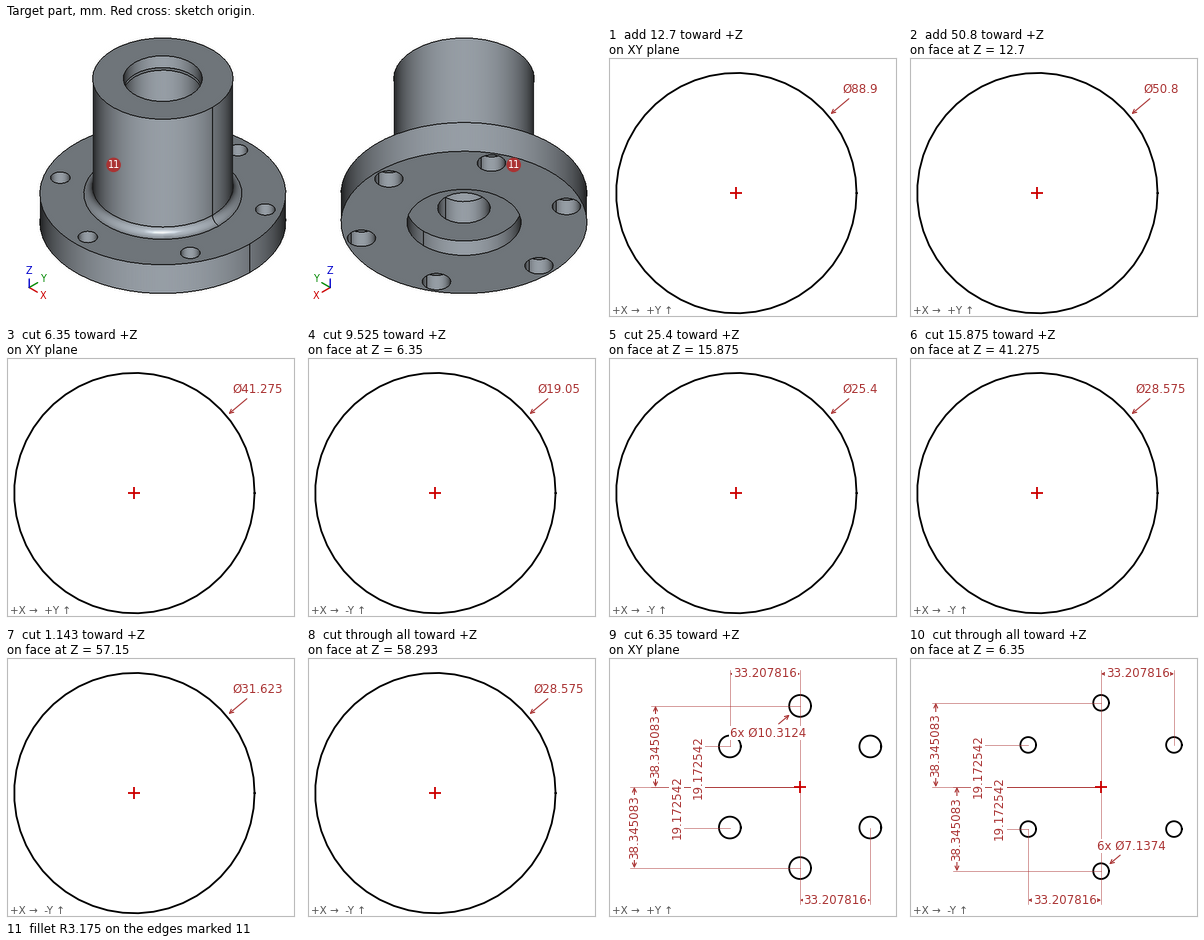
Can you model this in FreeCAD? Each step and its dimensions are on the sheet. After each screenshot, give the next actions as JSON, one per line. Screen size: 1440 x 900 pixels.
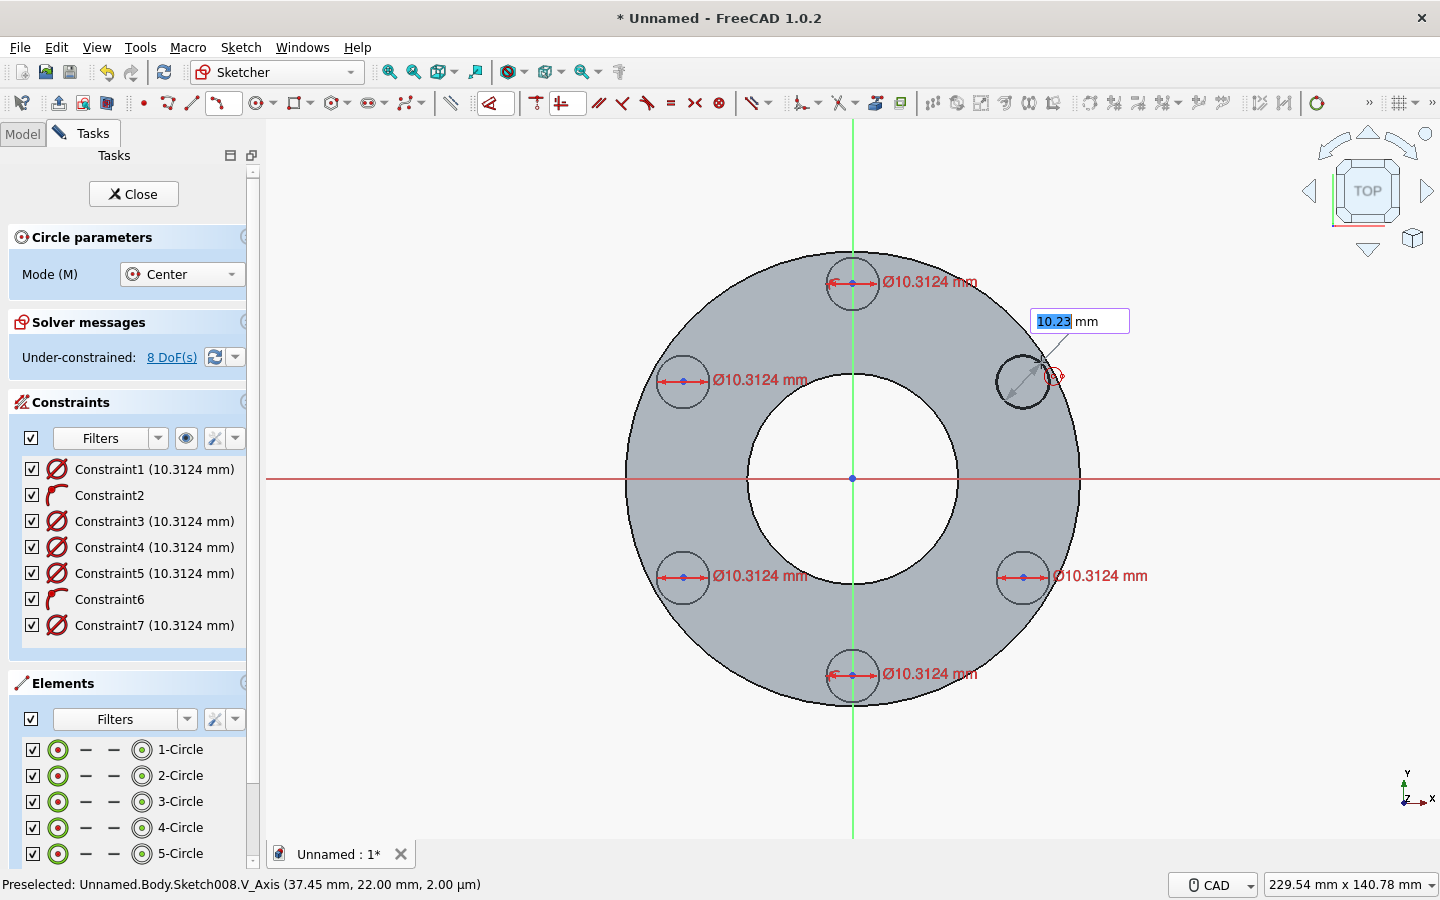
{"action": "type", "text": "10.3124"}
{"action": "key", "text": "Return"}
{"action": "key", "text": "Escape"}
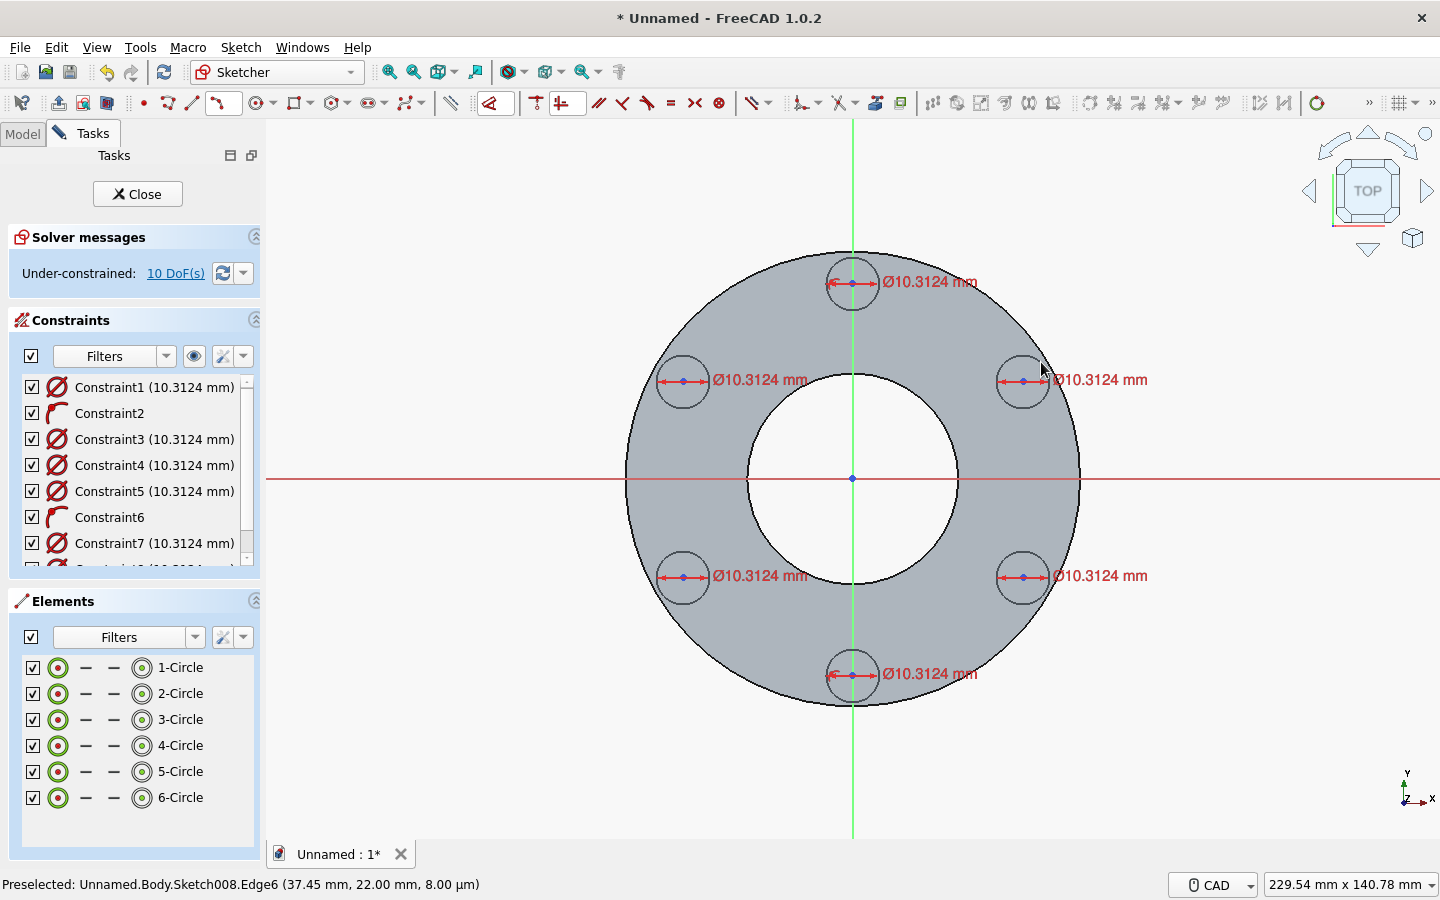
{"action": "left_click", "coordinate": [683, 382]}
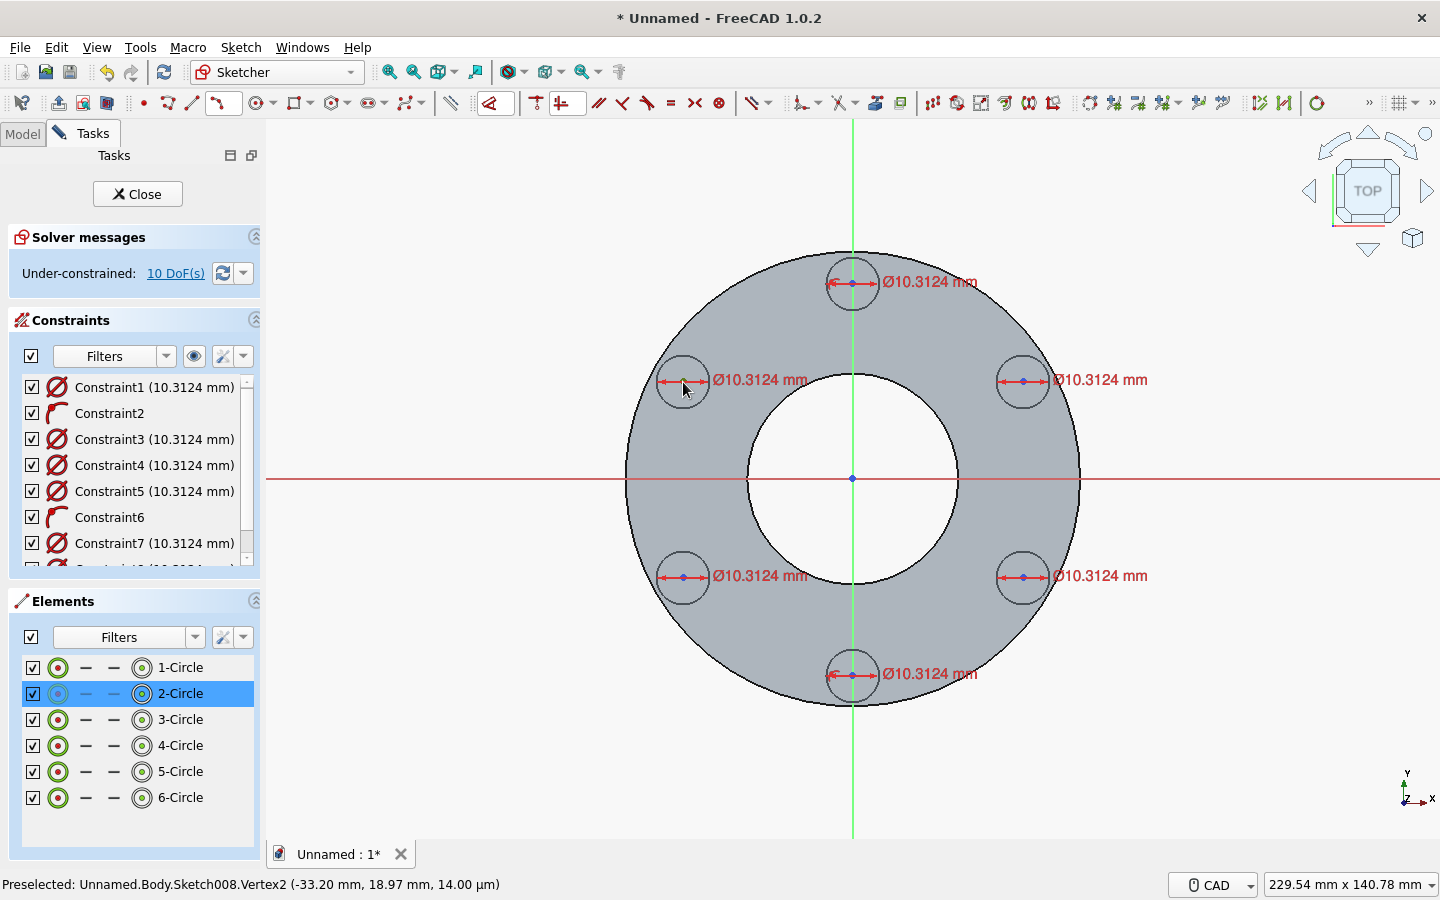
{"action": "left_click", "coordinate": [683, 578]}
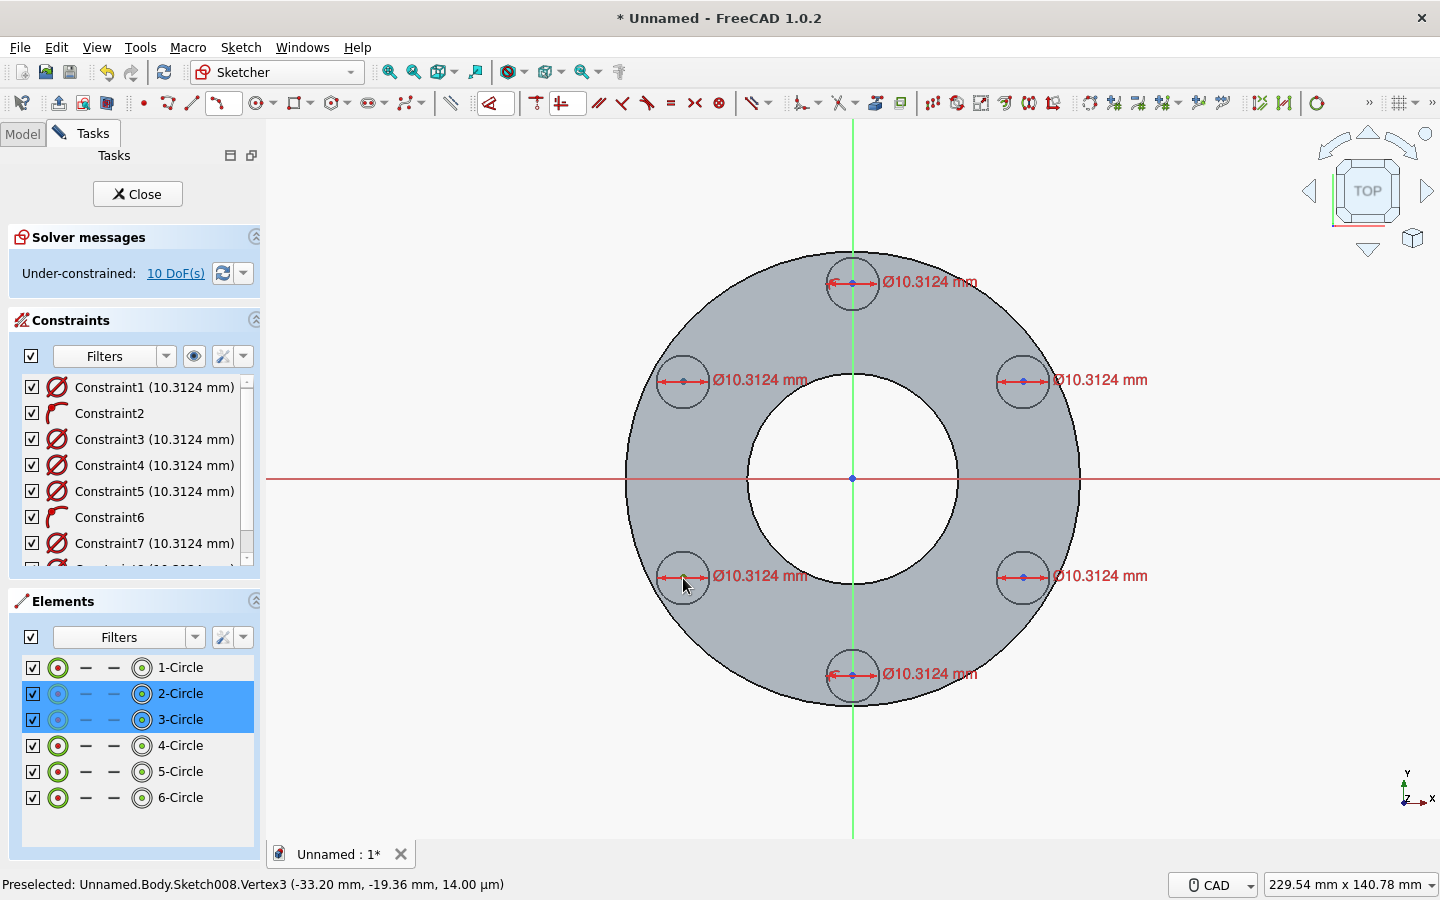
{"action": "key", "text": "v"}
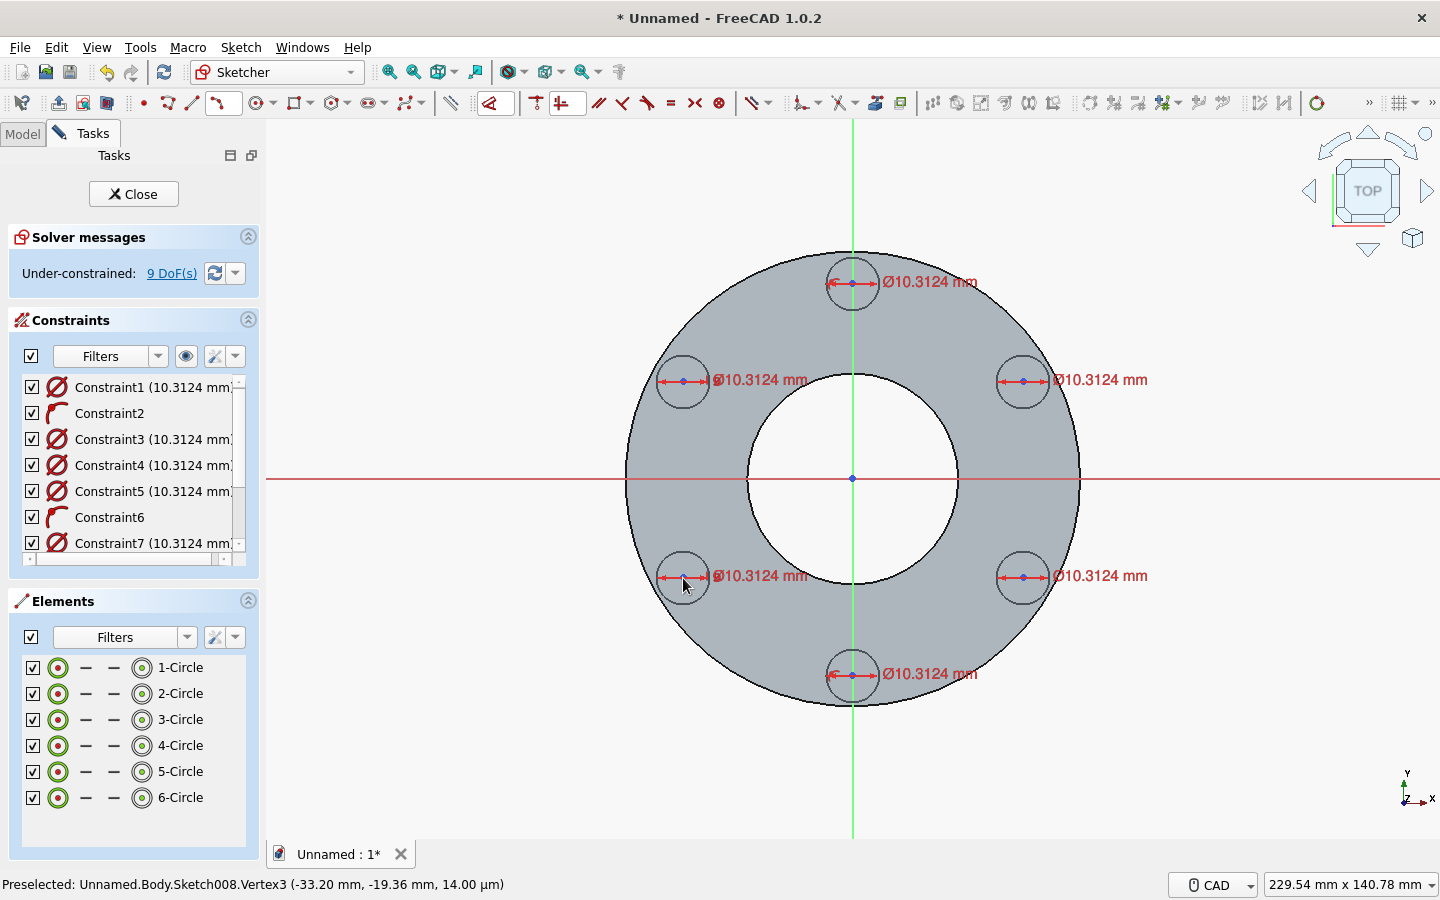
{"action": "left_click", "coordinate": [683, 578]}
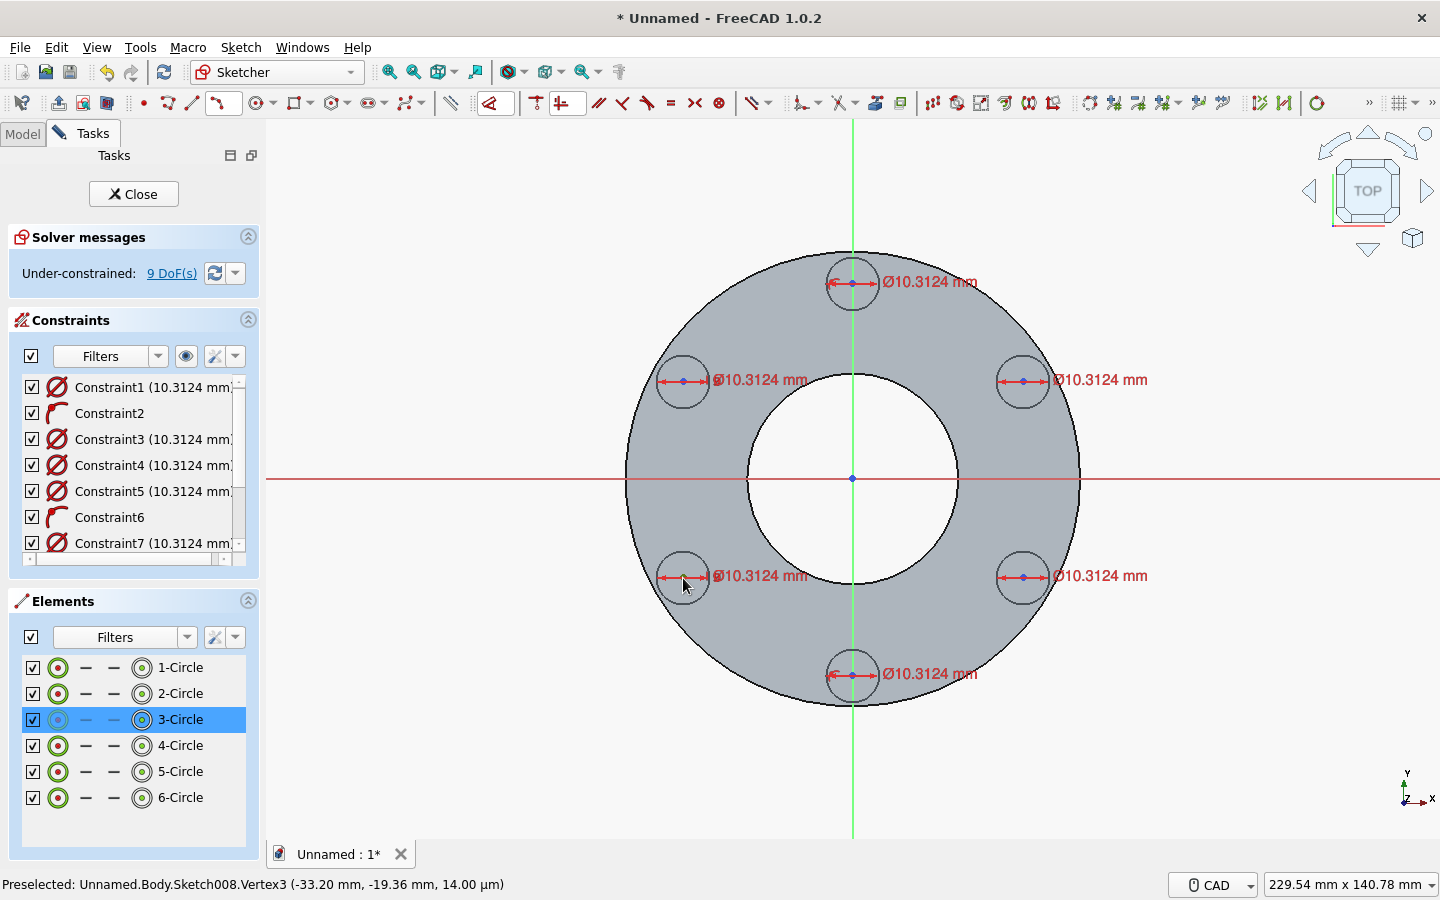
{"action": "left_click", "coordinate": [1023, 578]}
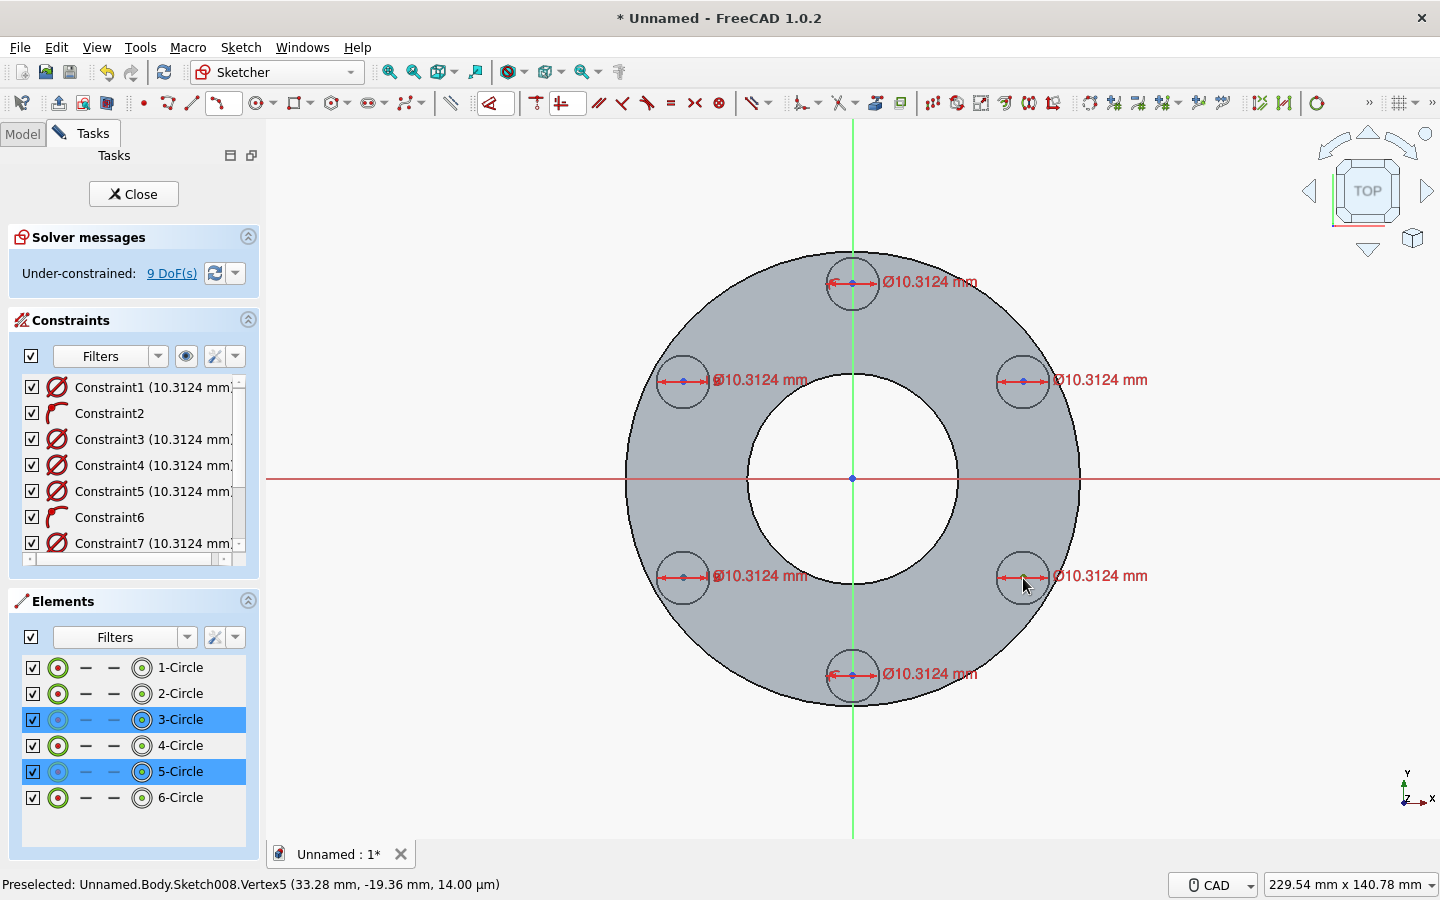
{"action": "key", "text": "h"}